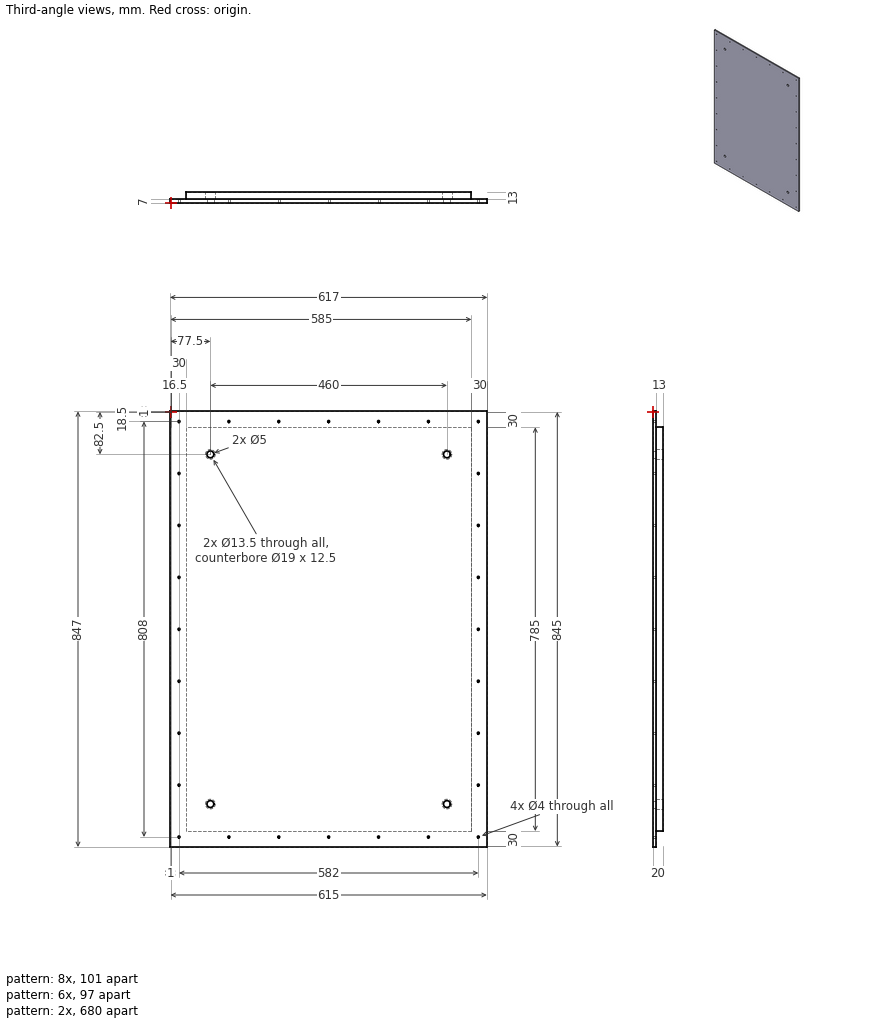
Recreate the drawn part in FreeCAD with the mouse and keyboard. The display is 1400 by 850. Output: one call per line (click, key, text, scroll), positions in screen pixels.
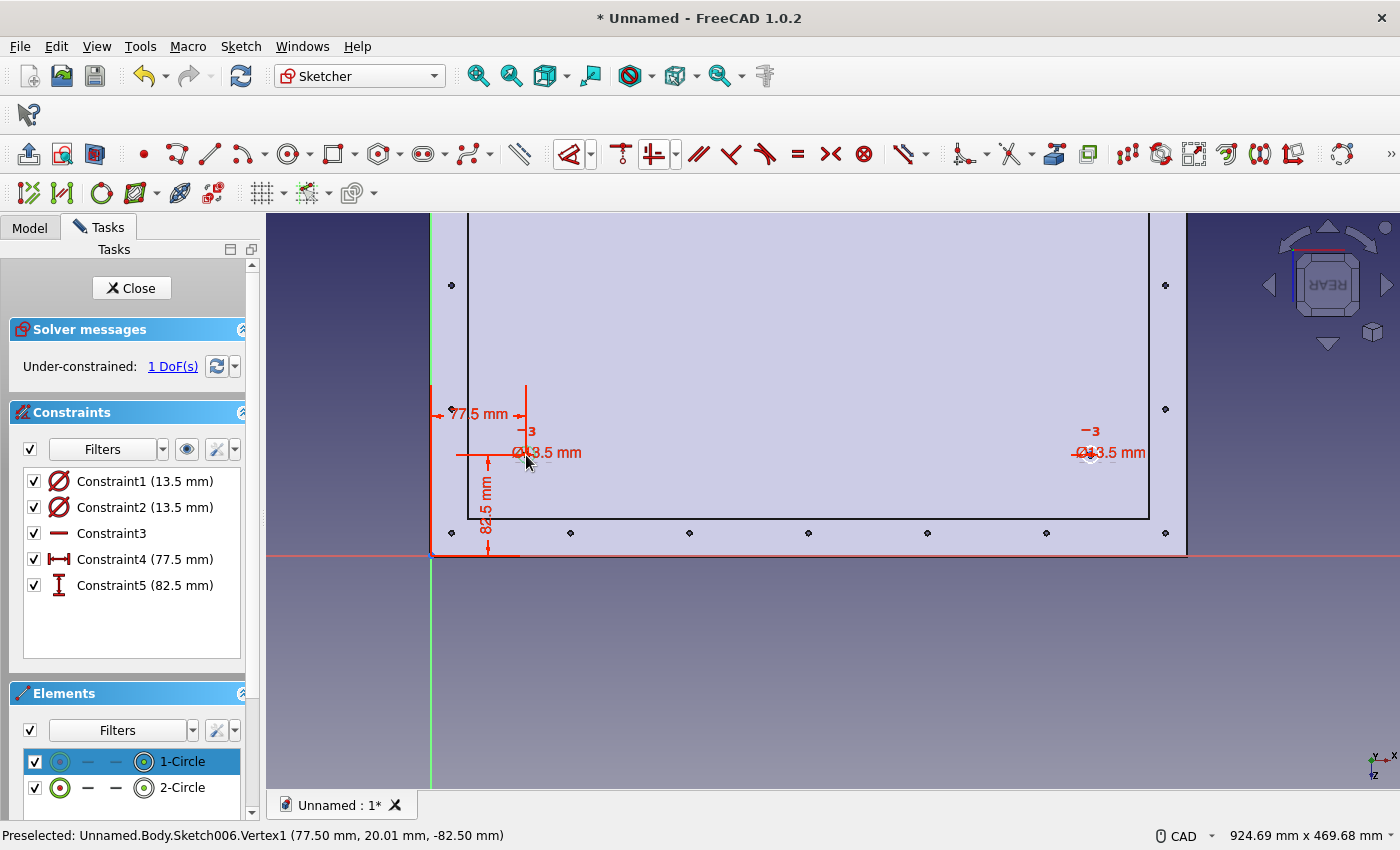
click(1091, 455)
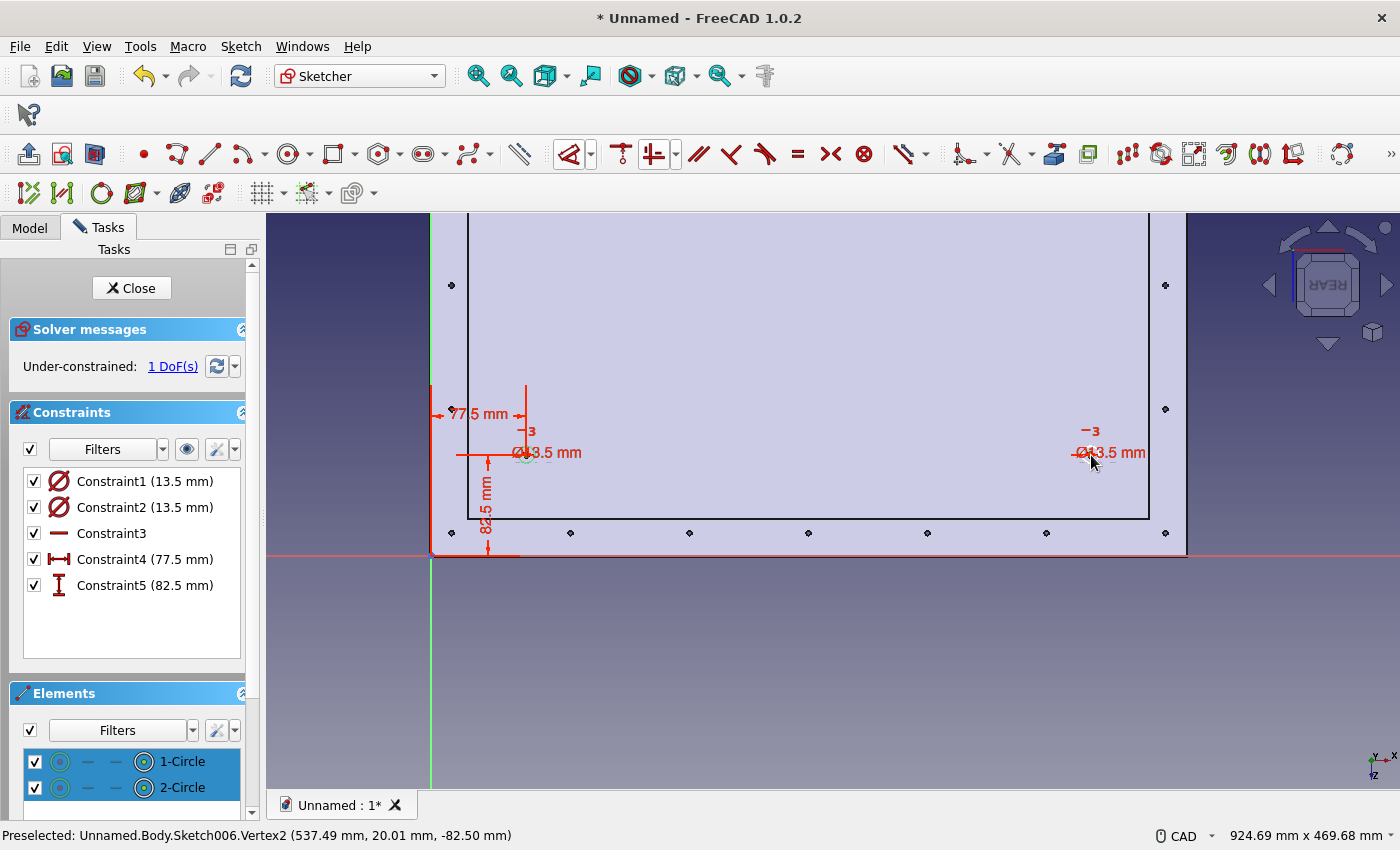
click(590, 154)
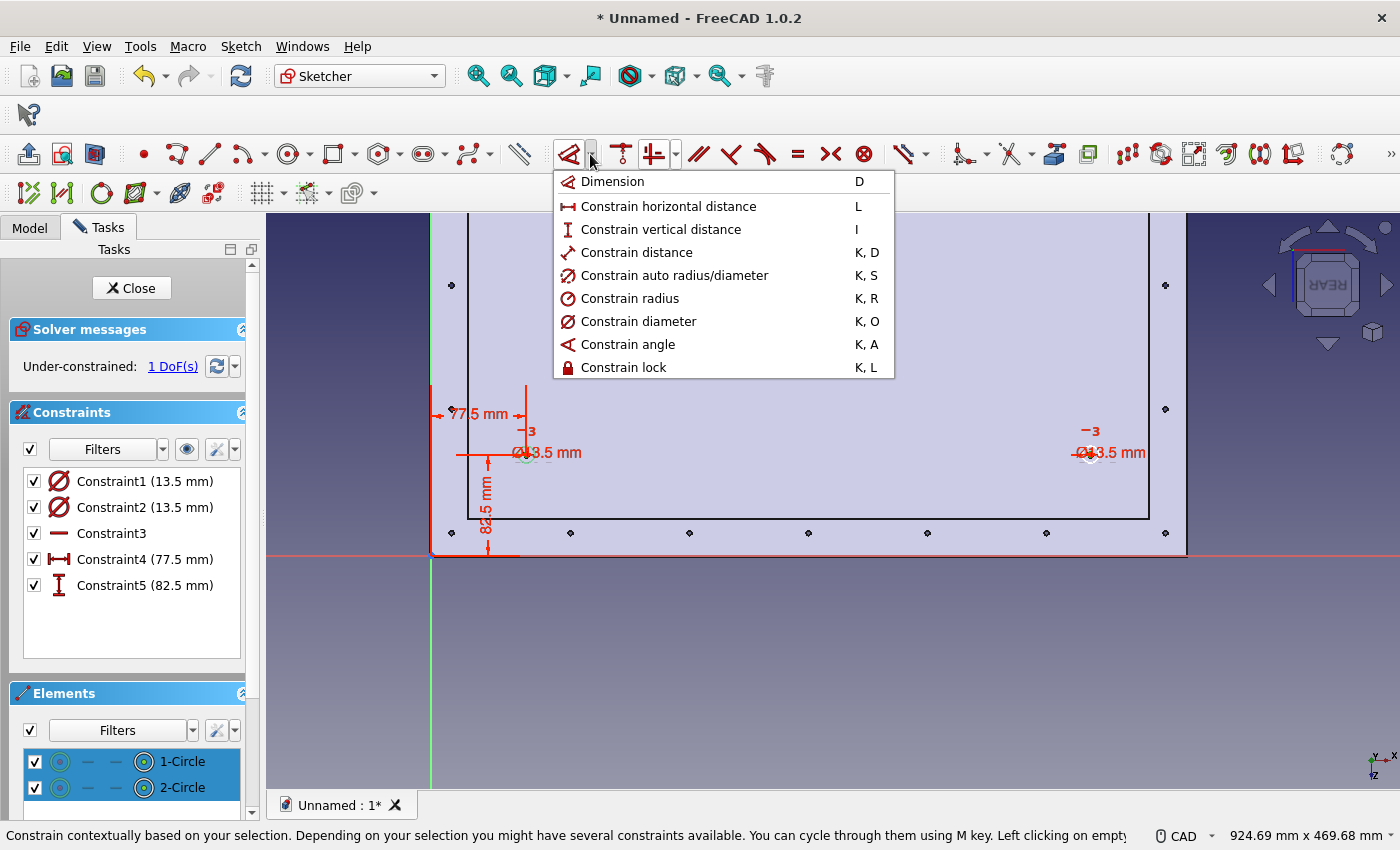
click(724, 206)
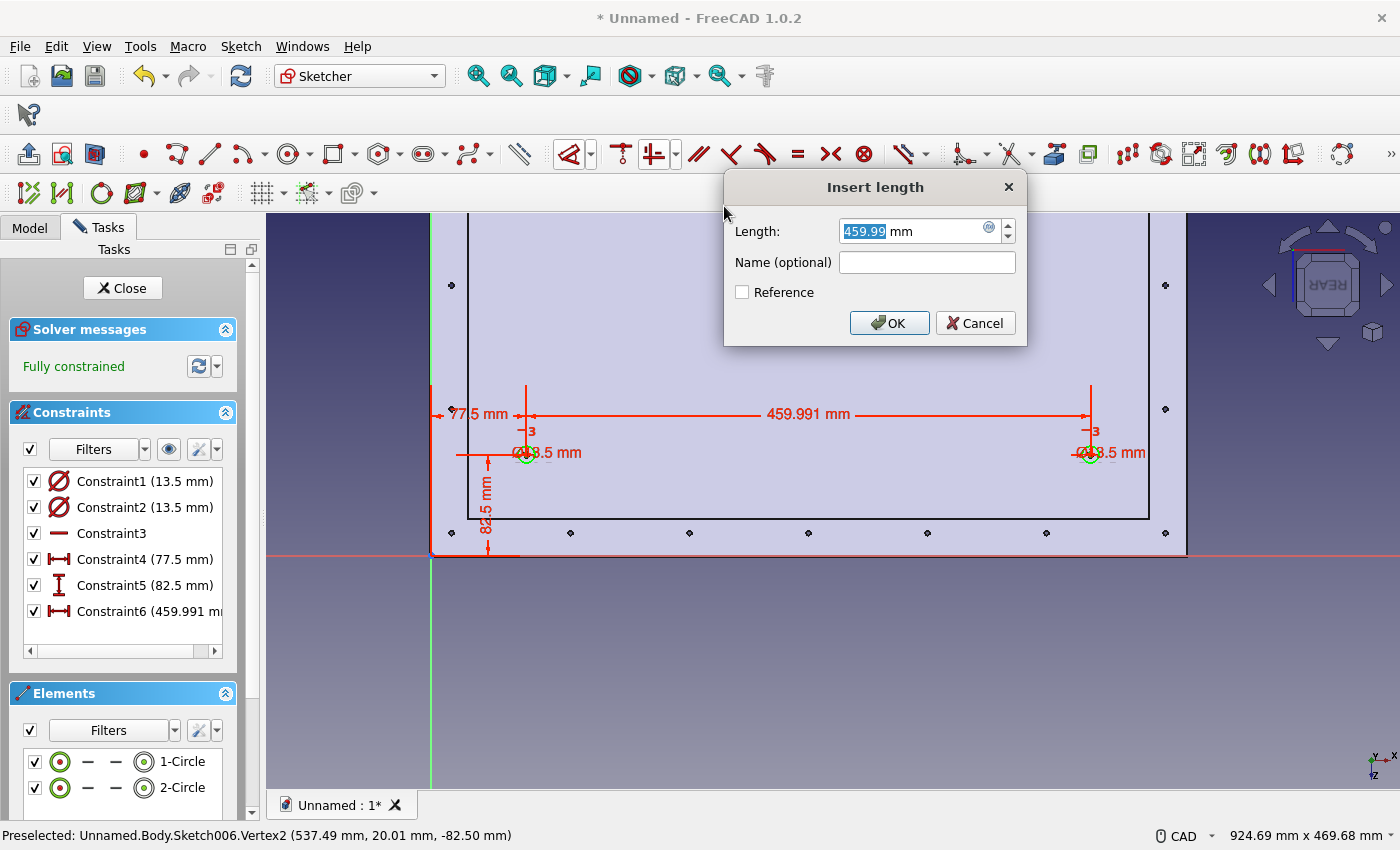
text(460)
key(Return)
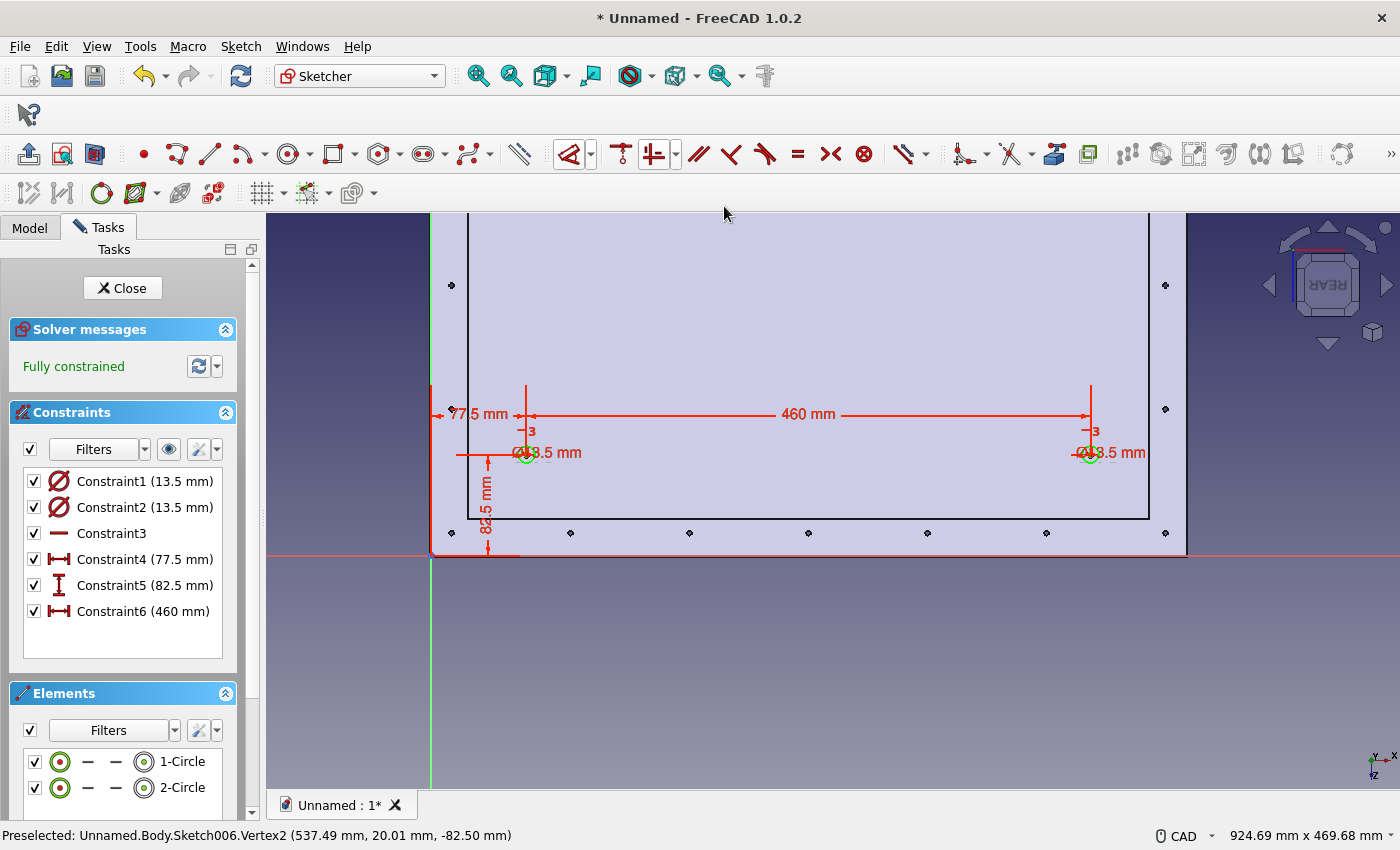
click(123, 288)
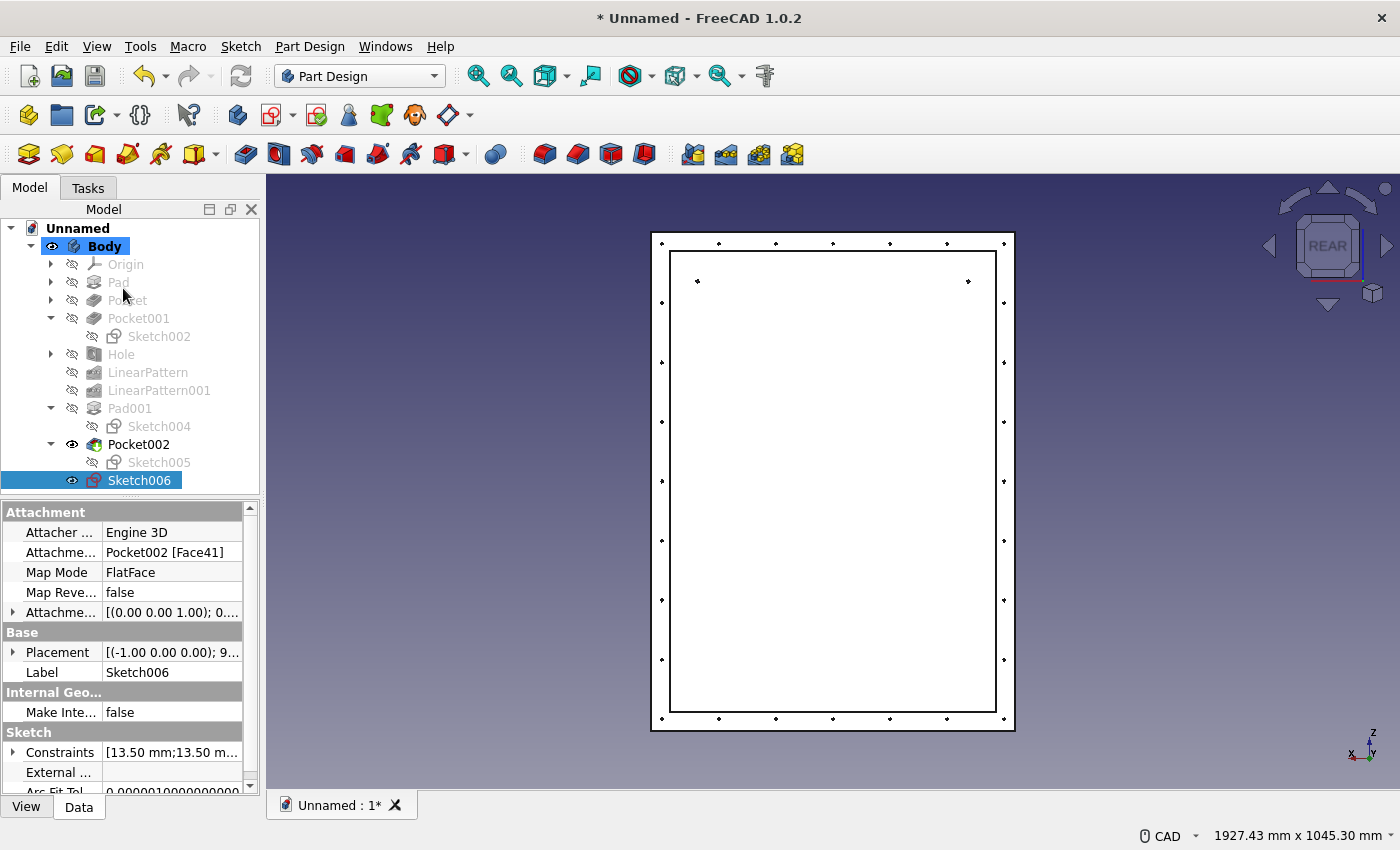
click(279, 154)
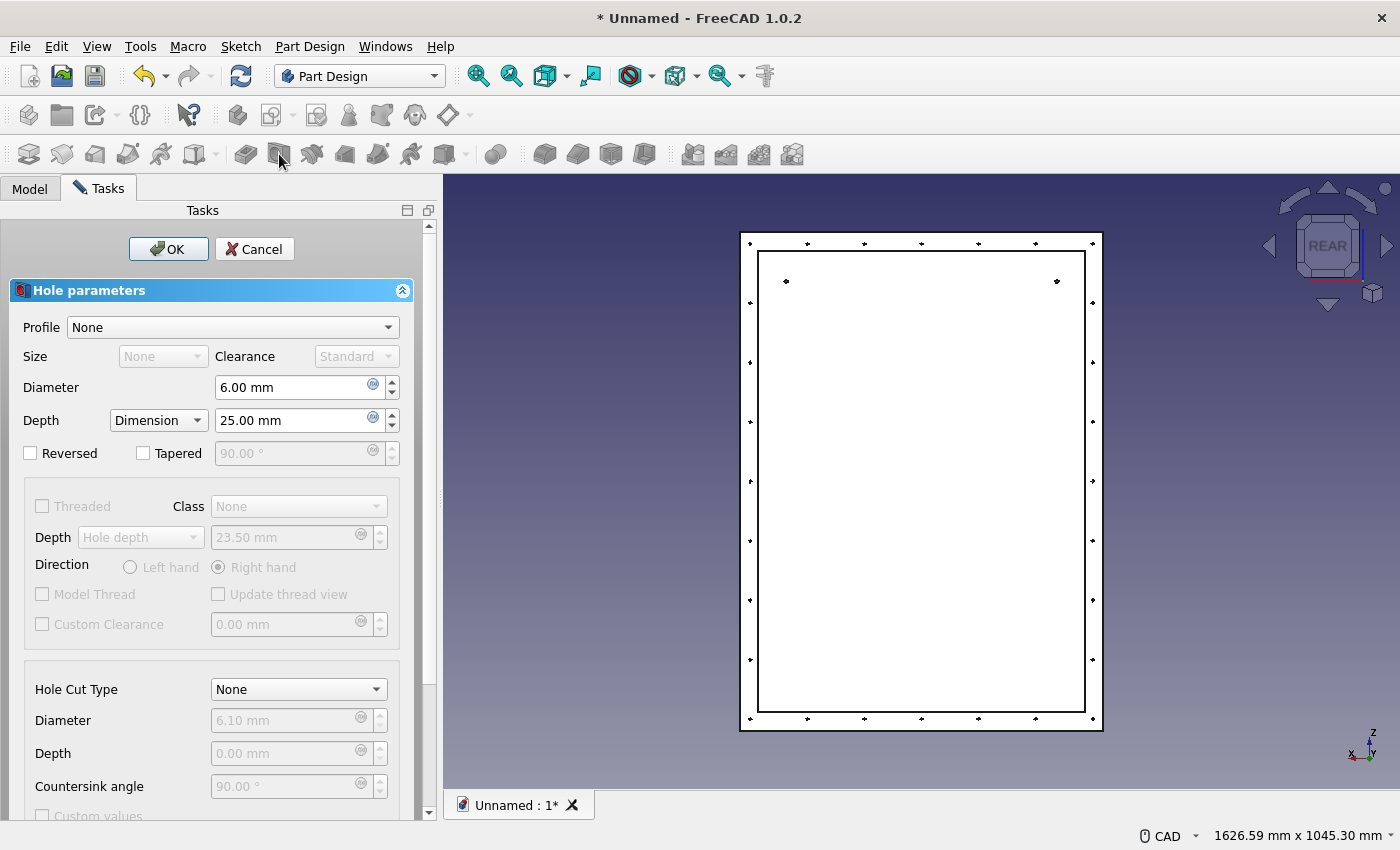
triple_click(300, 388)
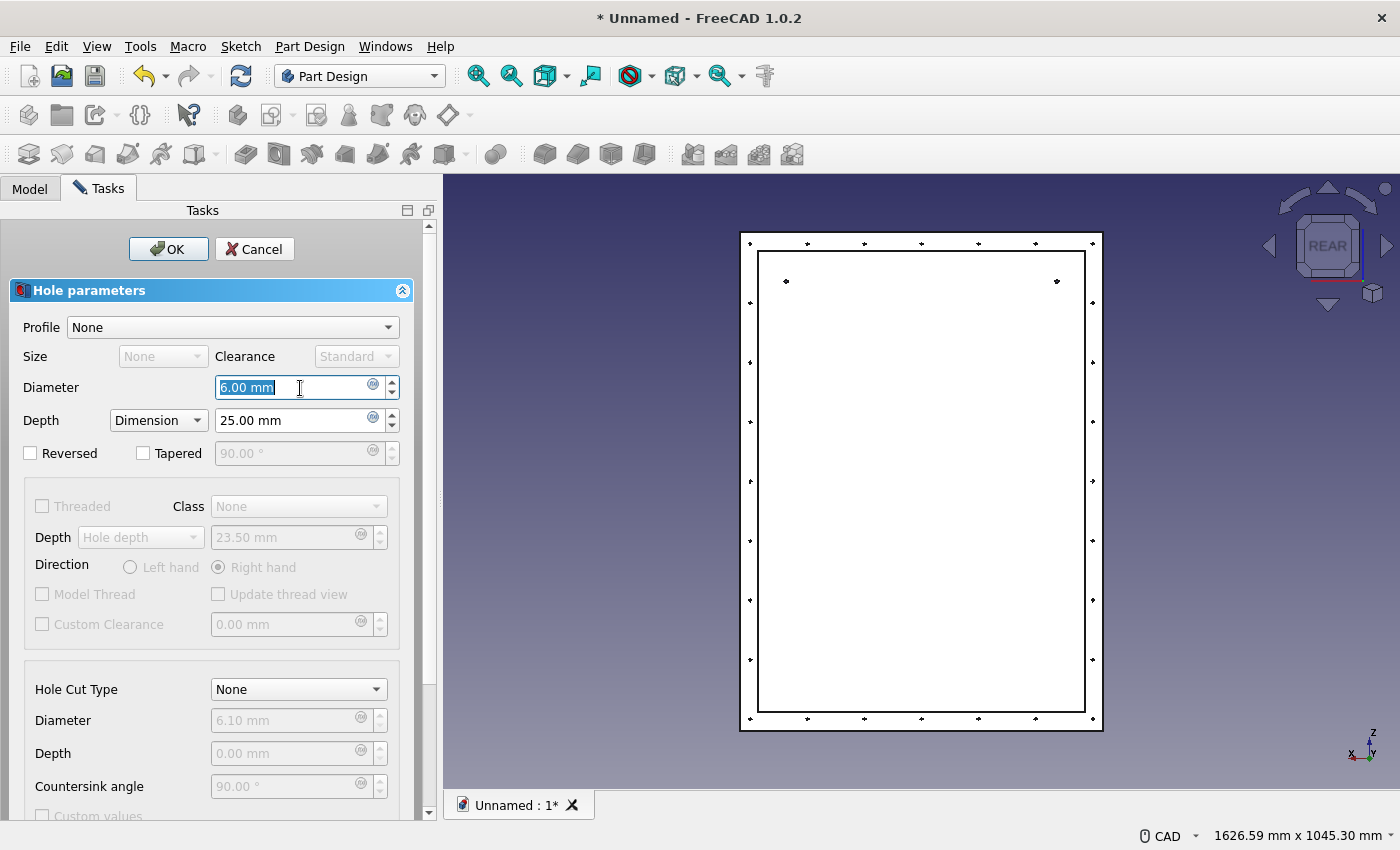
text(13.5)
key(Tab)